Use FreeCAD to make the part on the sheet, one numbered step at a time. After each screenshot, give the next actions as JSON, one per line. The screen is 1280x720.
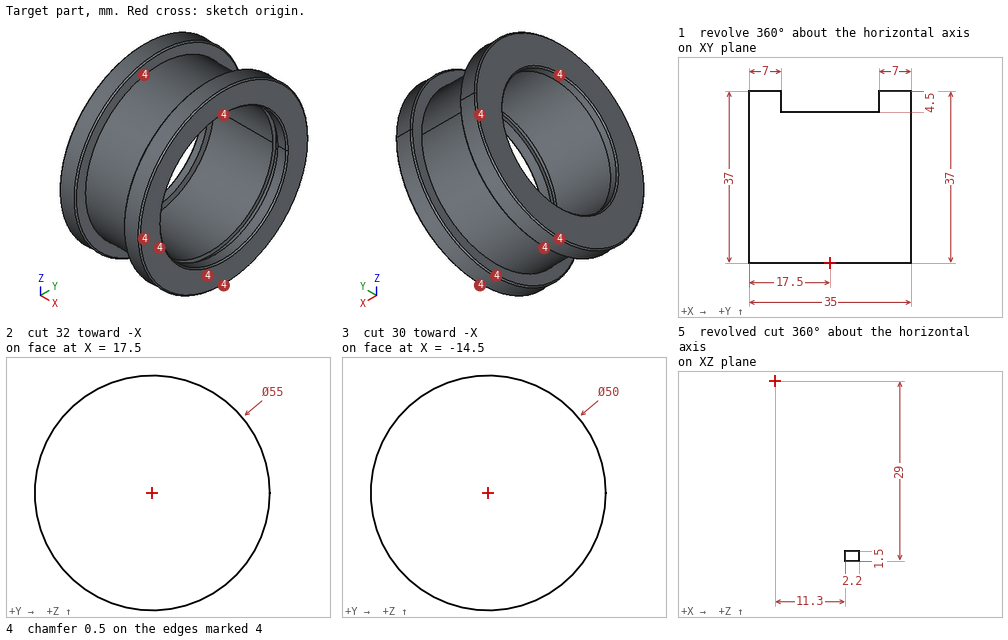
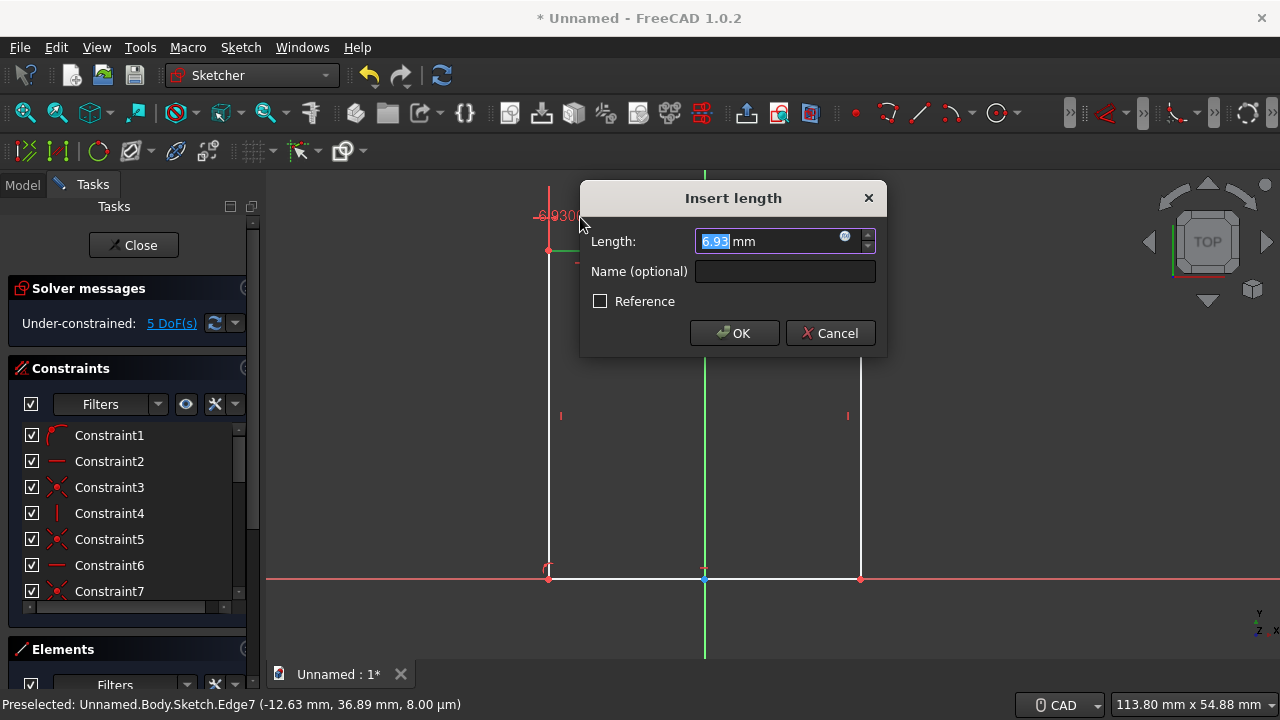
{"action": "type", "text": "7"}
{"action": "key", "text": "Return"}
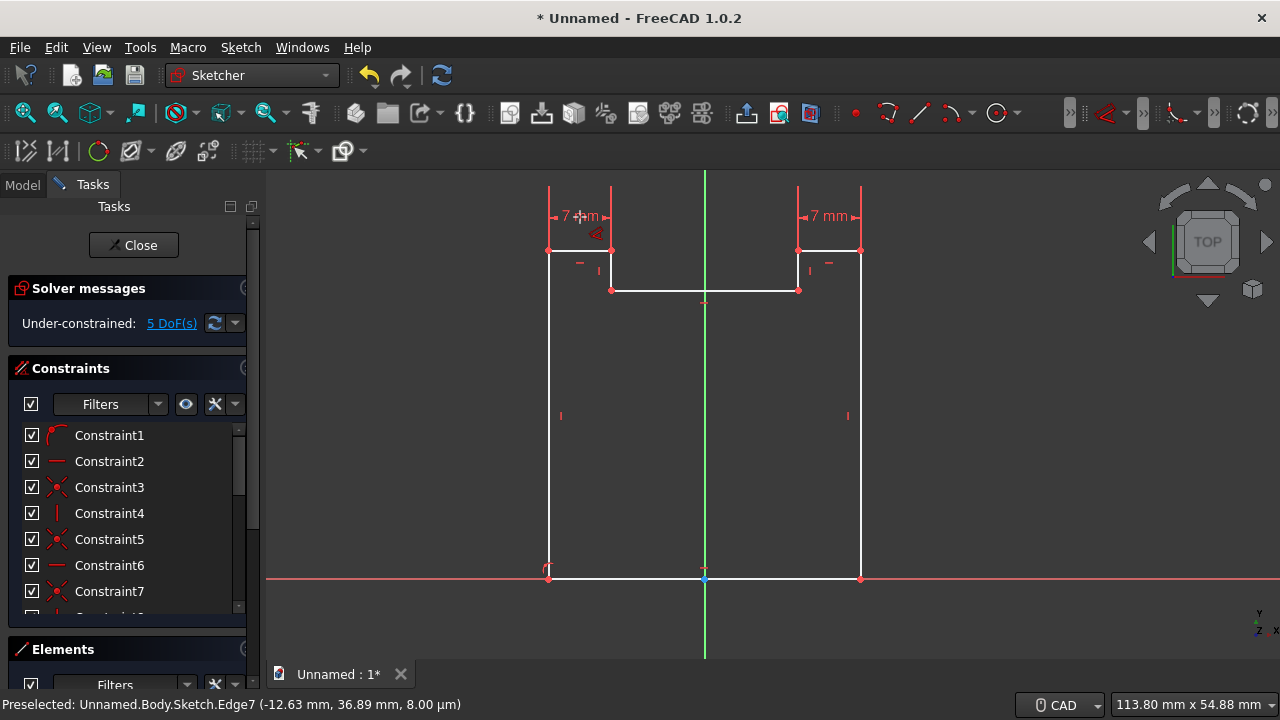
{"action": "left_click", "coordinate": [642, 579]}
{"action": "left_click", "coordinate": [633, 613]}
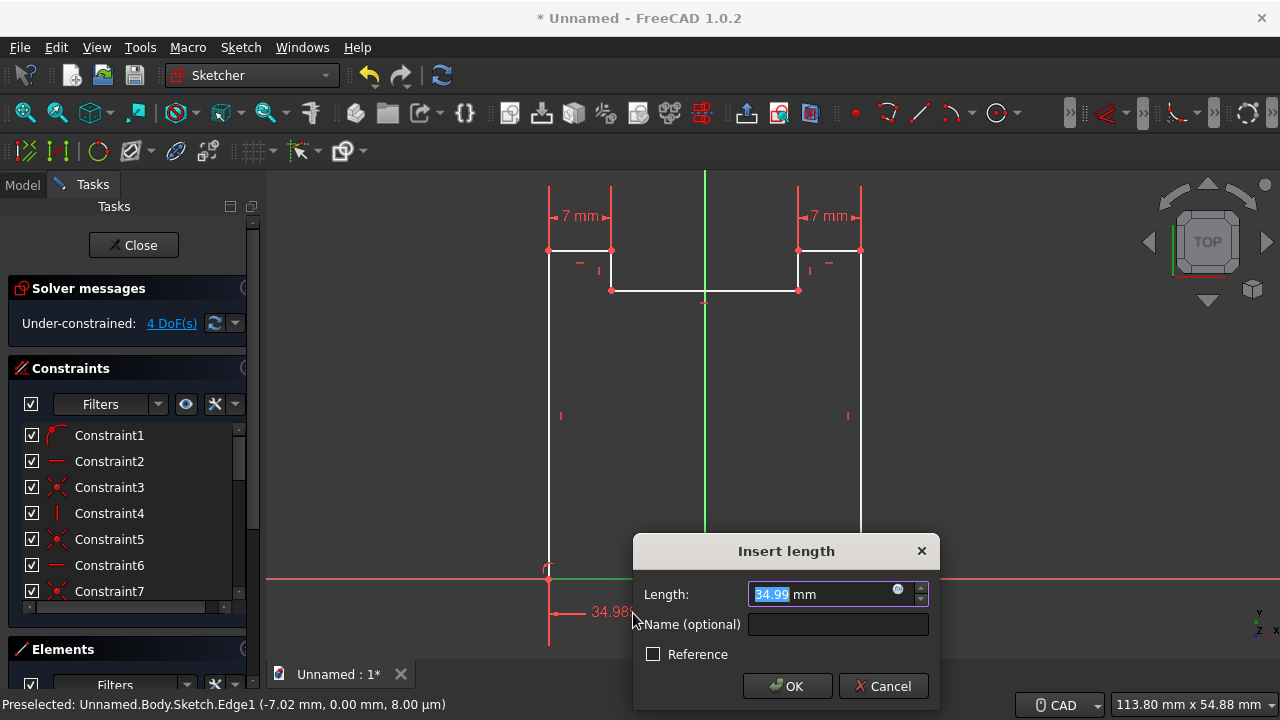
{"action": "type", "text": "35"}
{"action": "key", "text": "Return"}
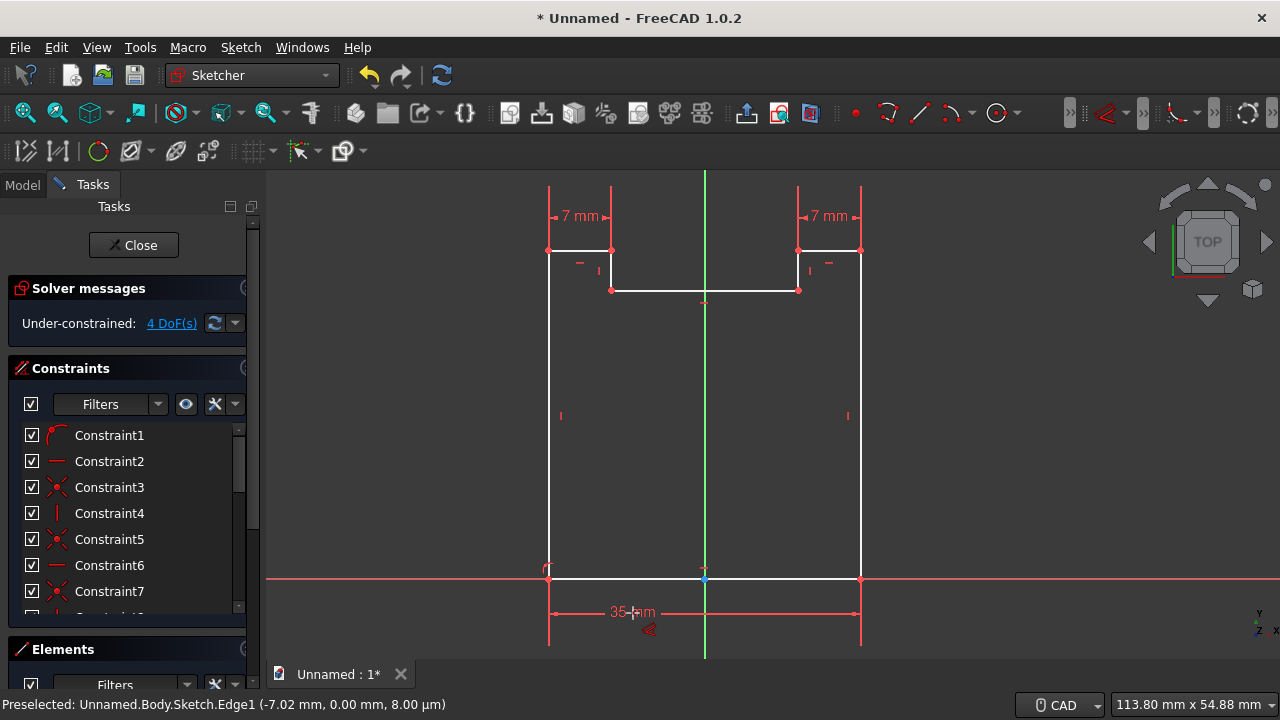
{"action": "left_click", "coordinate": [861, 481]}
{"action": "left_click", "coordinate": [895, 415]}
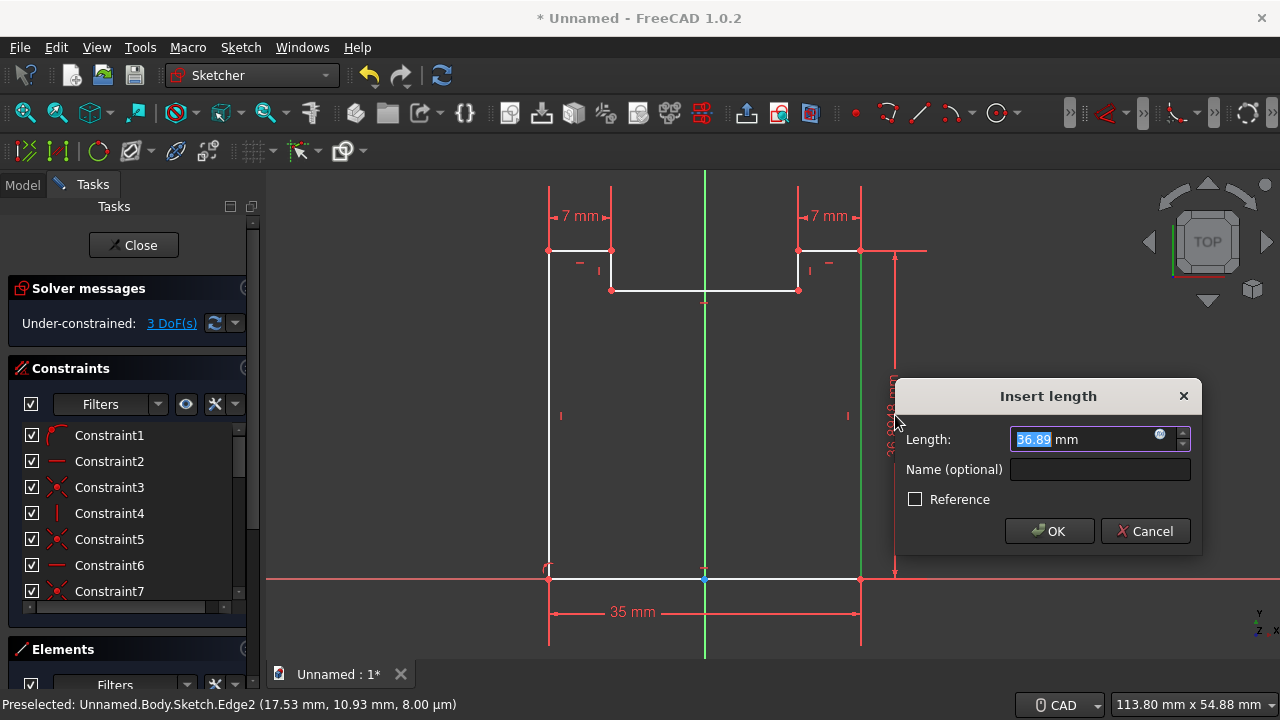
{"action": "type", "text": "37"}
{"action": "key", "text": "Return"}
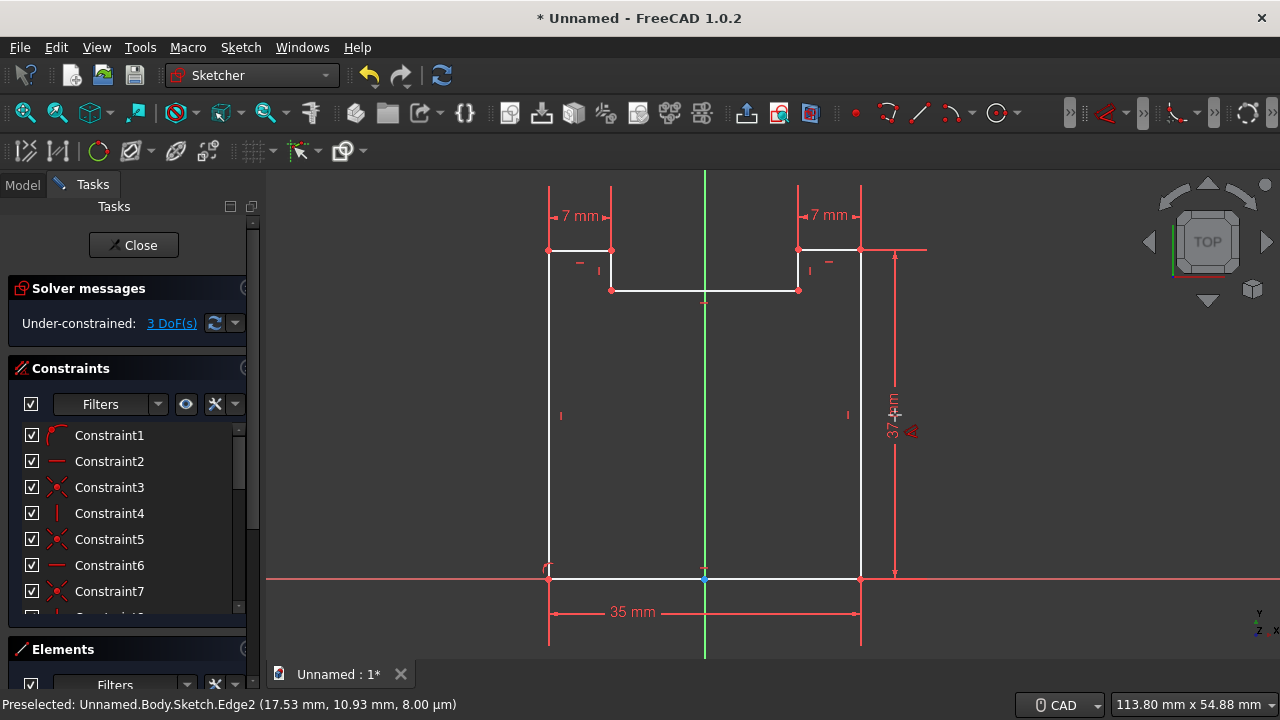
{"action": "left_click", "coordinate": [549, 349]}
{"action": "left_click", "coordinate": [515, 415]}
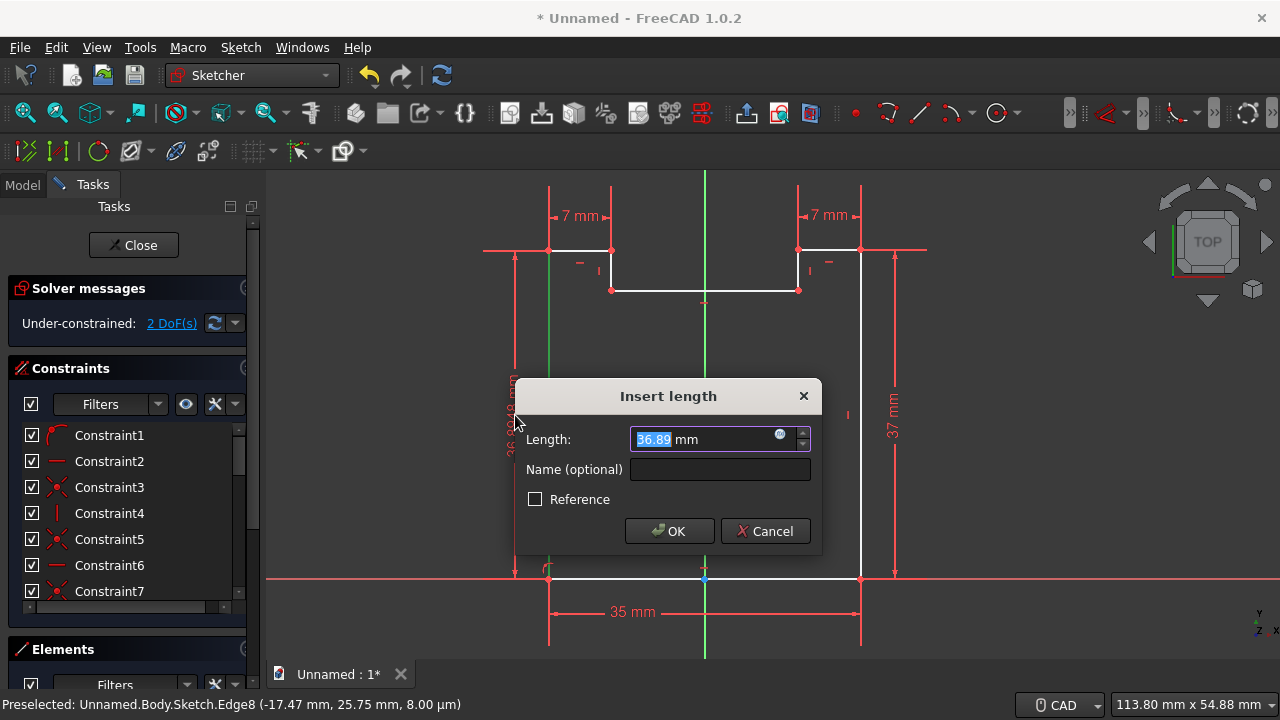
{"action": "type", "text": "37"}
{"action": "key", "text": "Return"}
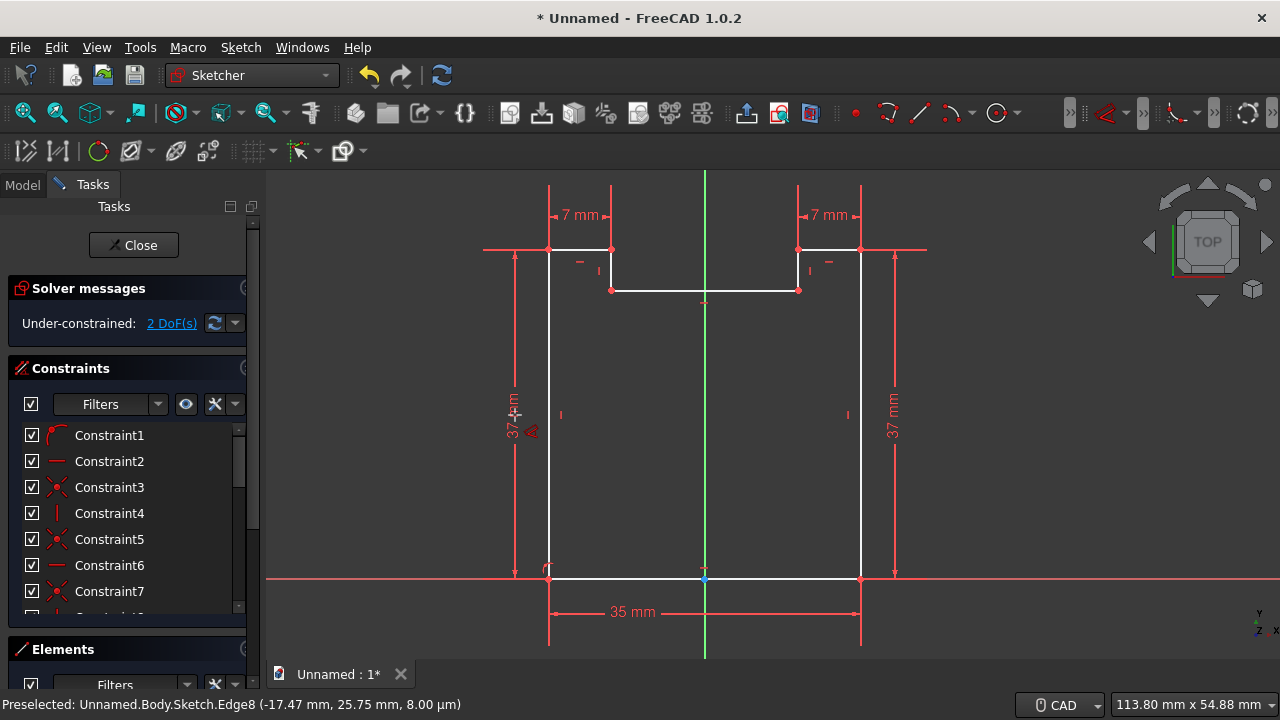
{"action": "left_click", "coordinate": [798, 262]}
{"action": "left_click", "coordinate": [832, 270]}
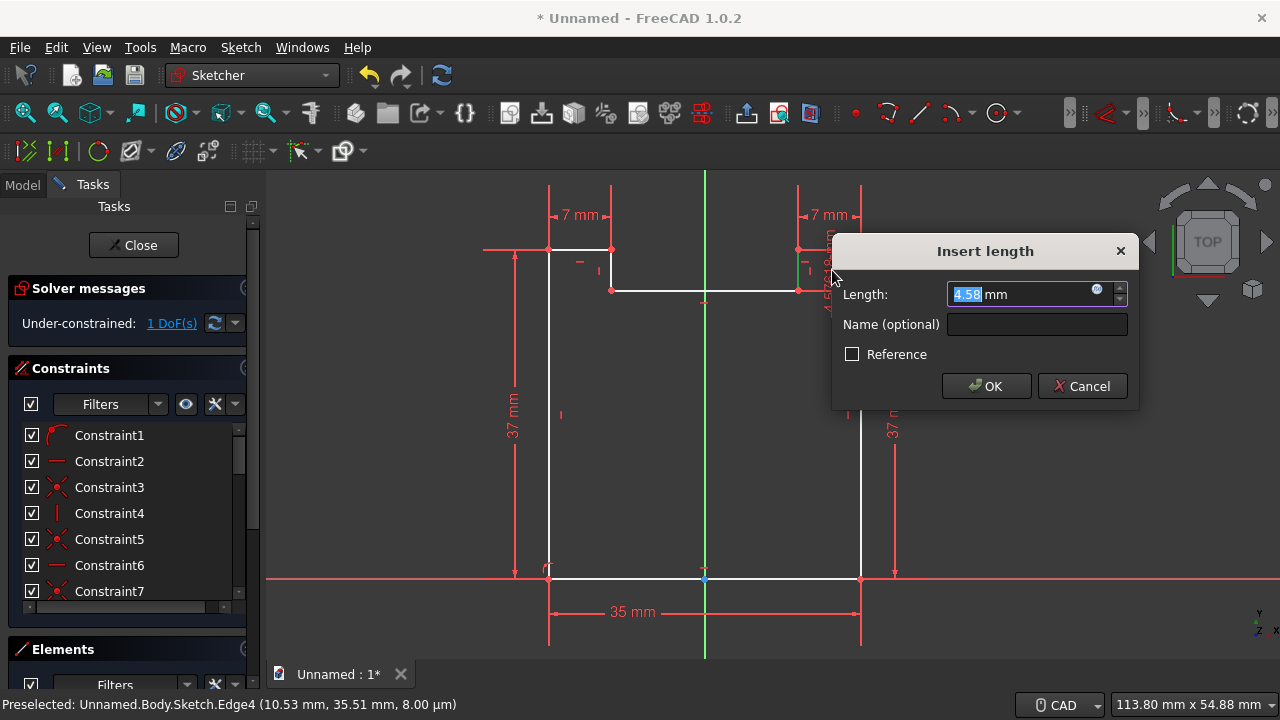
{"action": "type", "text": "4.5"}
{"action": "key", "text": "Return"}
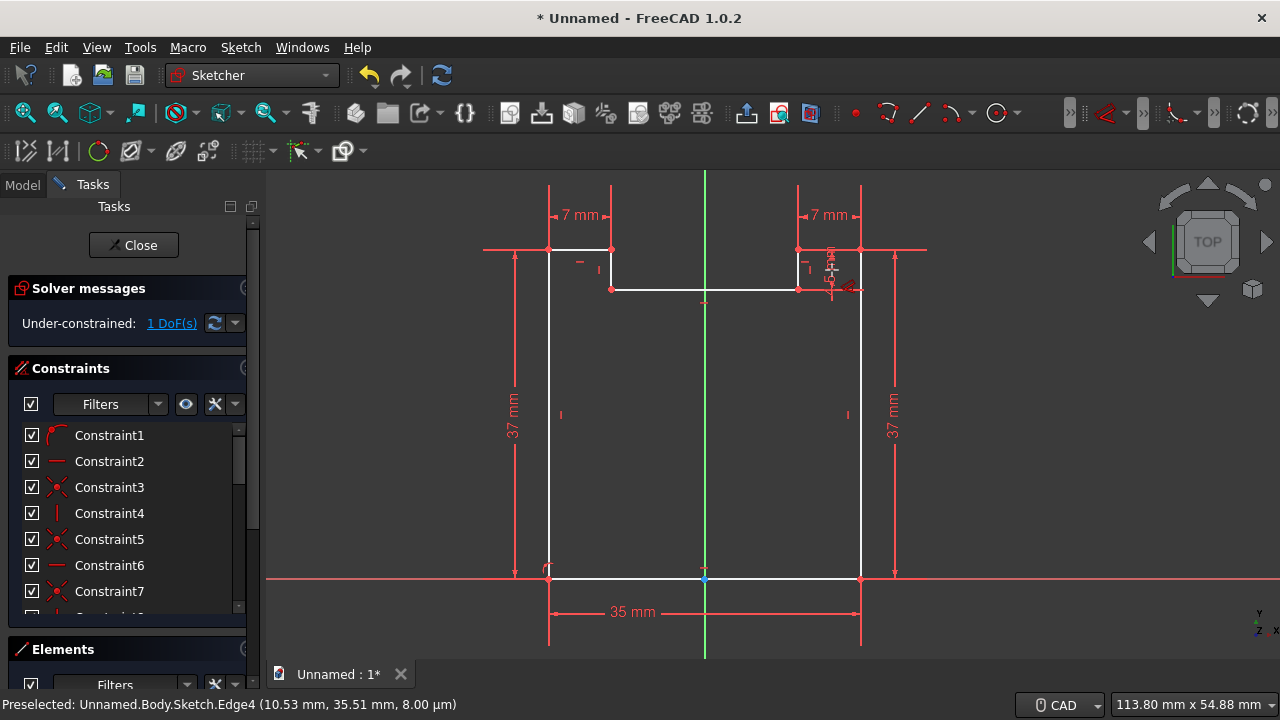
{"action": "left_click", "coordinate": [549, 579]}
{"action": "left_click", "coordinate": [627, 545]}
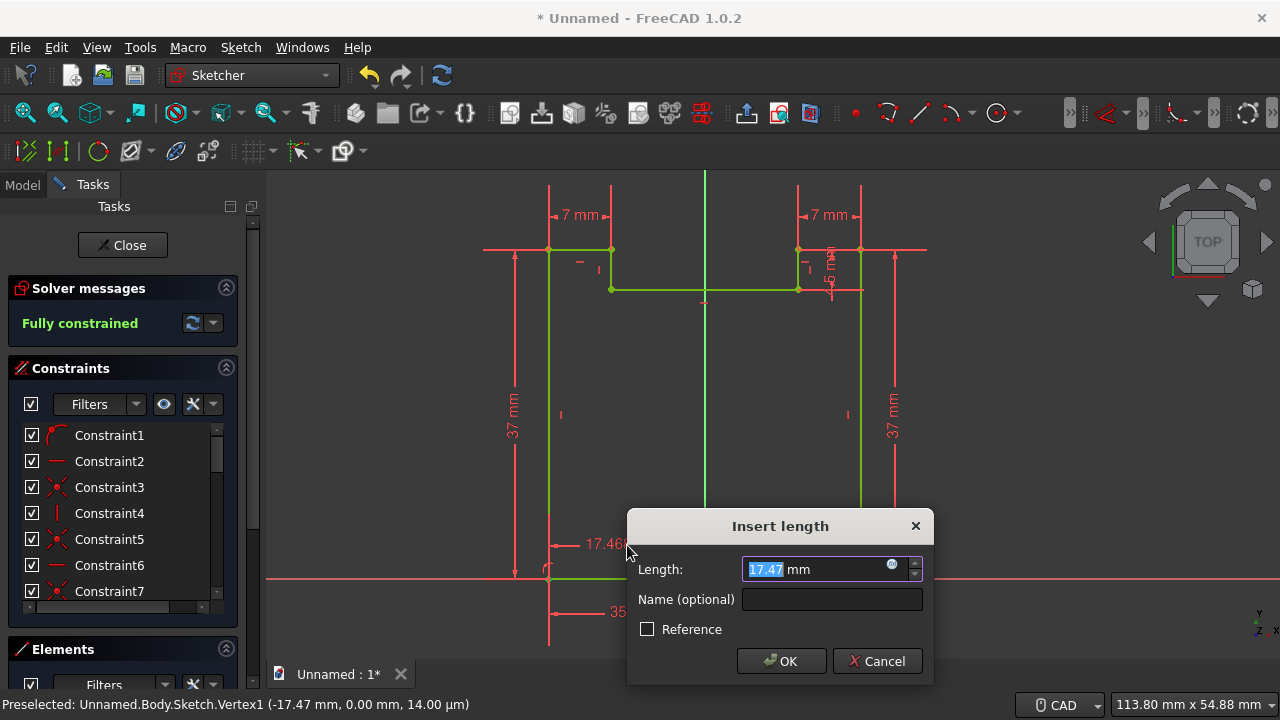
{"action": "type", "text": "17.5"}
{"action": "key", "text": "Return"}
{"action": "key", "text": "Escape"}